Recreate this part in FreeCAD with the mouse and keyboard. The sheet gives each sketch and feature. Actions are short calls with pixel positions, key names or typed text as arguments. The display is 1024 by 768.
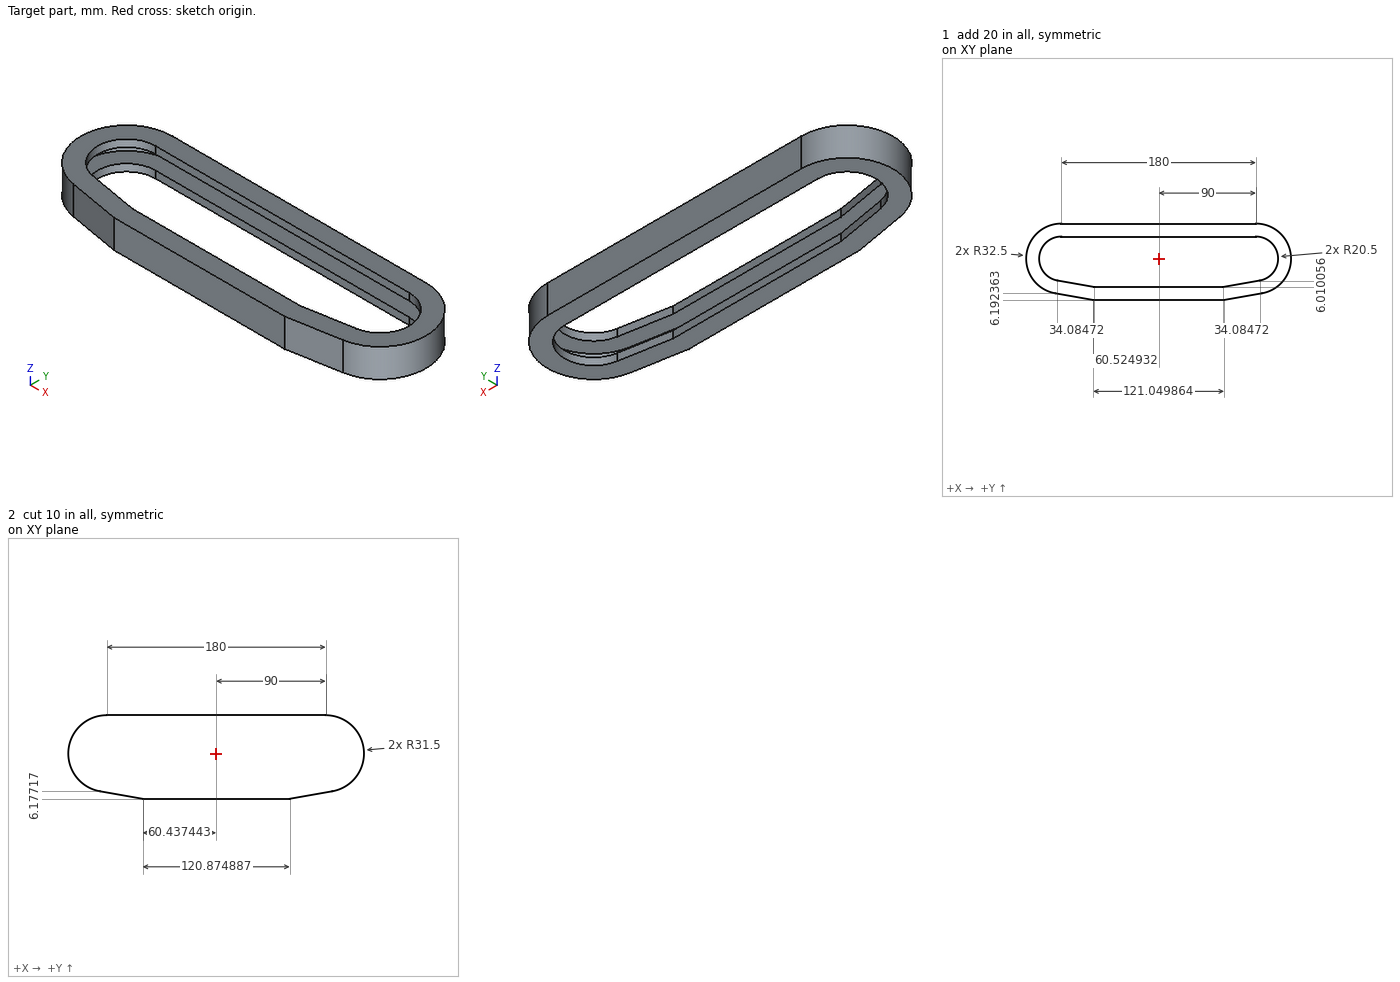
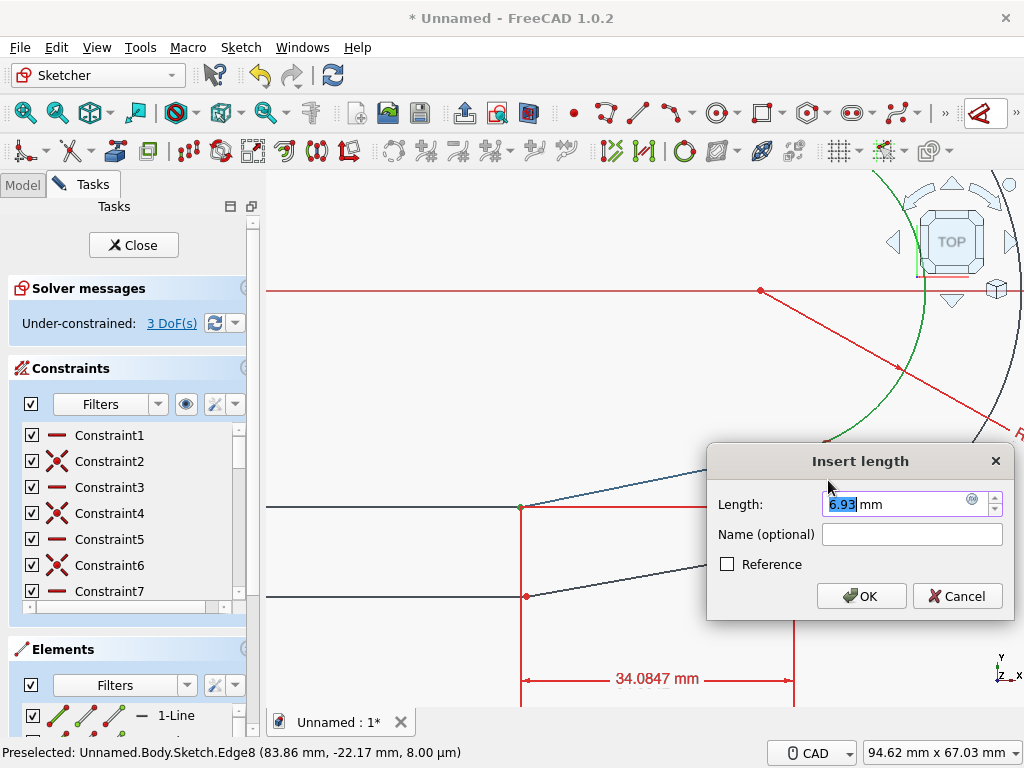
text(6.010056)
key(Return)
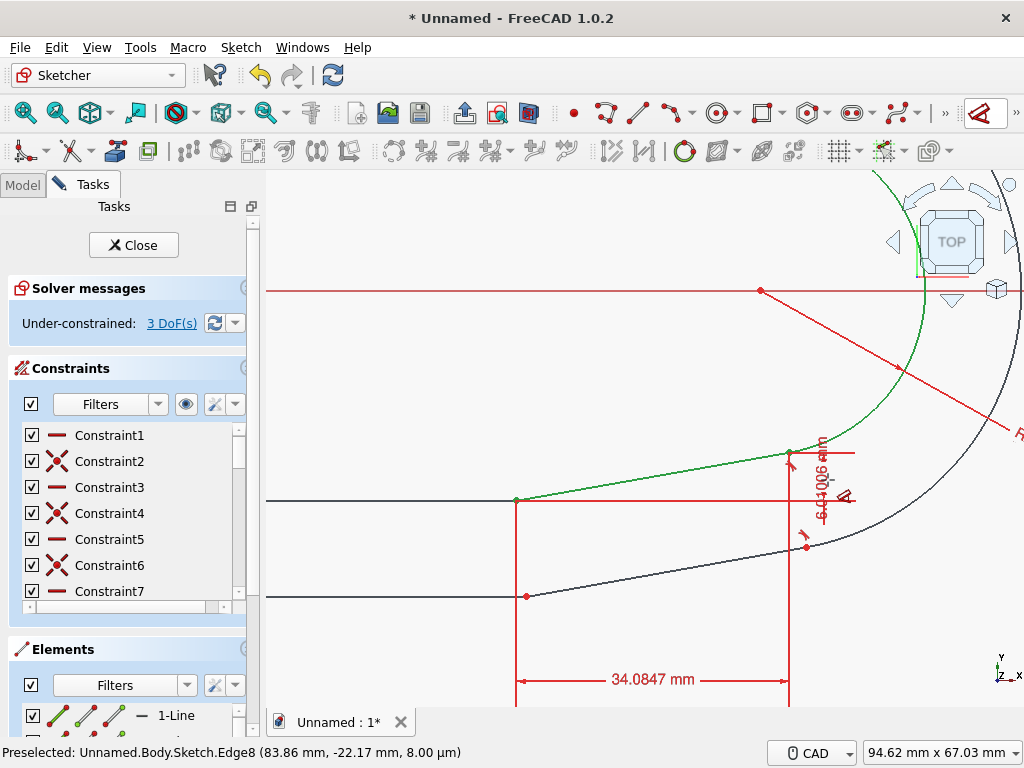
scroll(712, 470, down, 8)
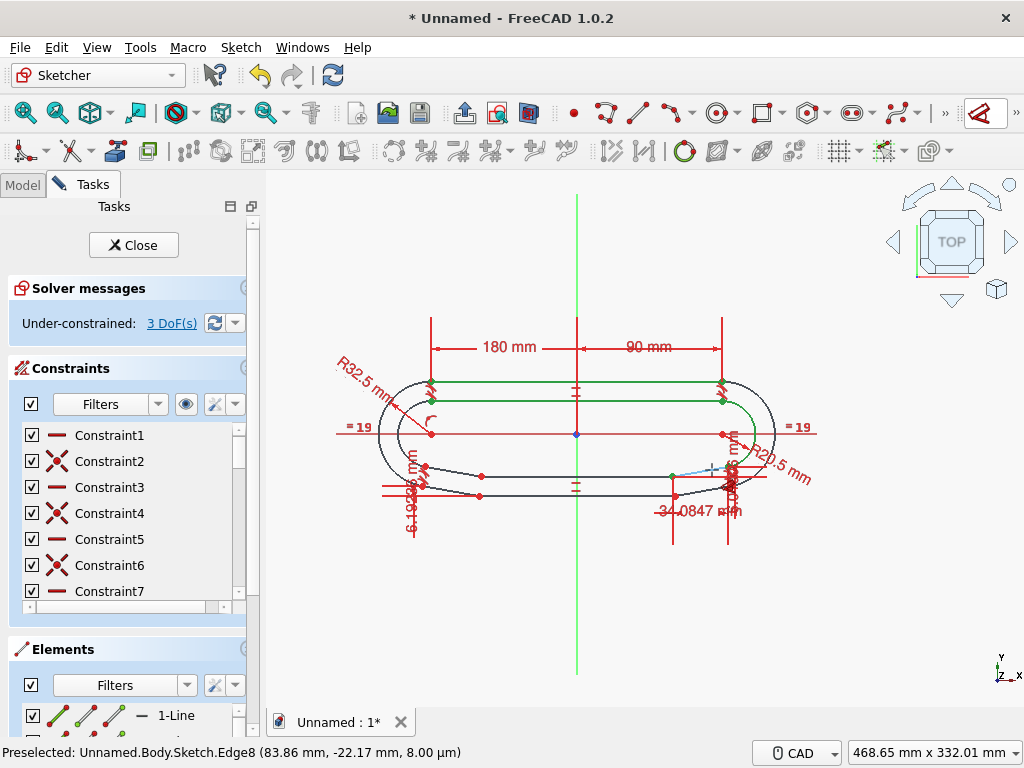
click(464, 474)
click(453, 535)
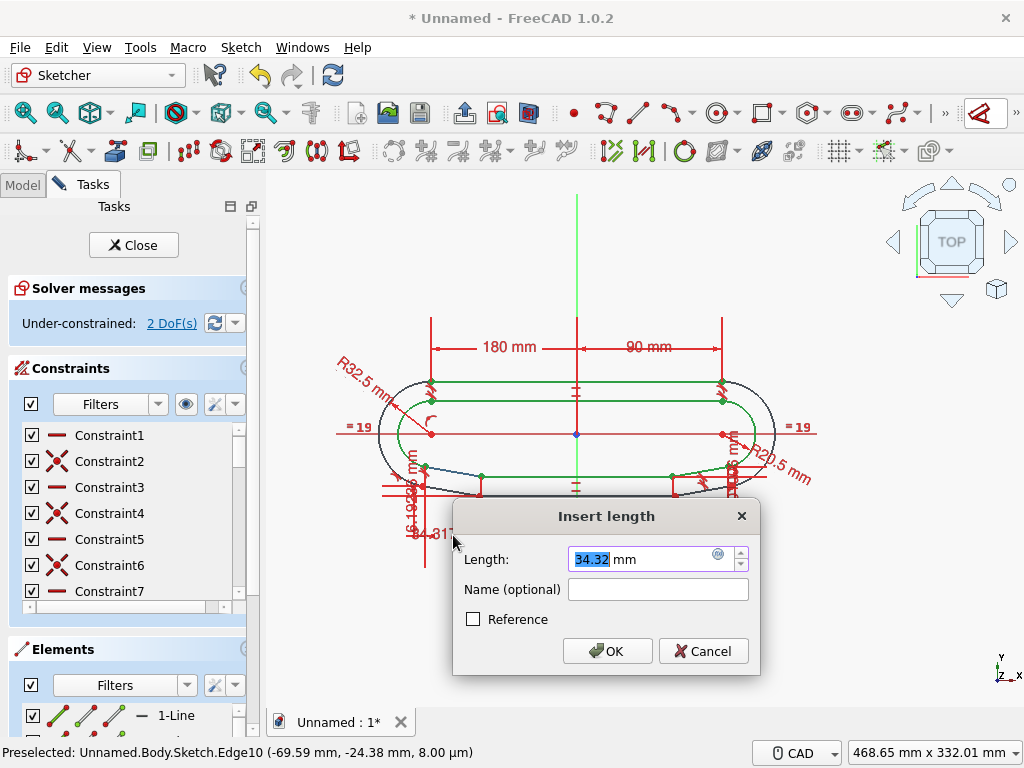
text(34.08472)
key(Return)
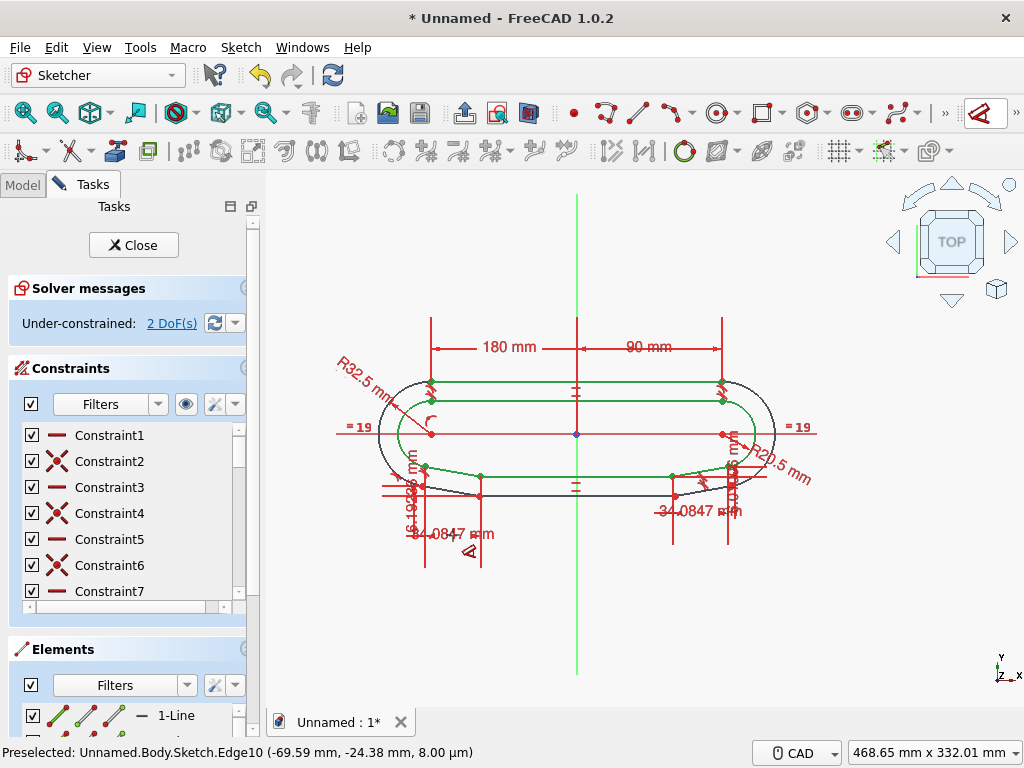
click(538, 496)
click(532, 530)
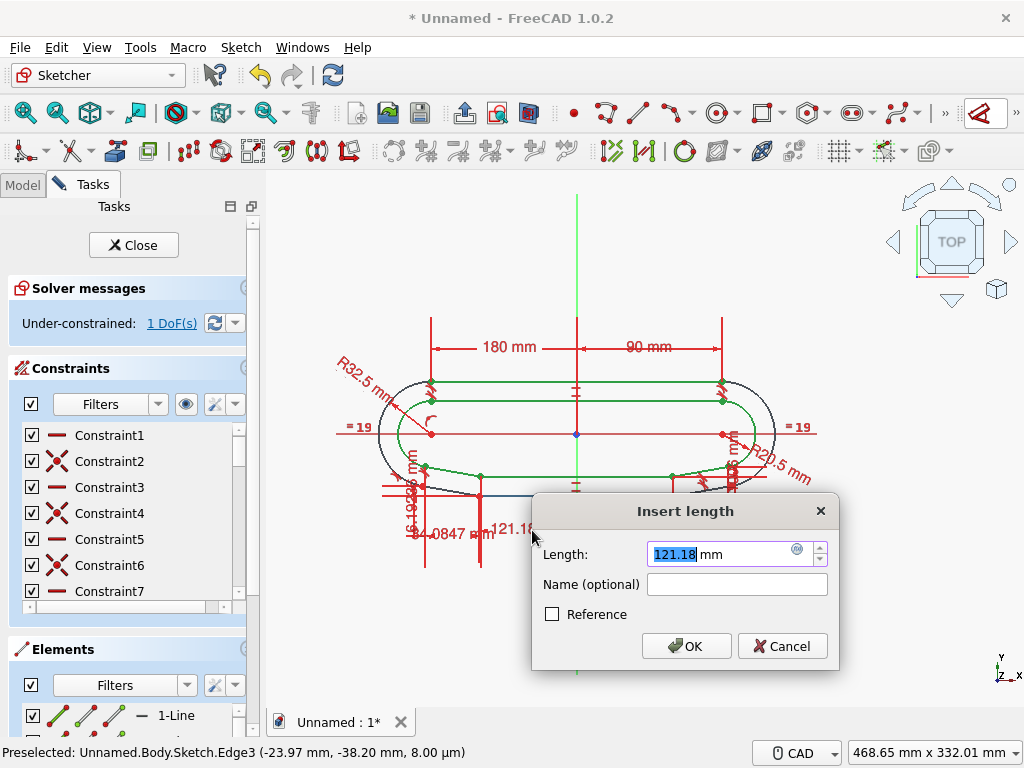
text(121.049864)
key(Return)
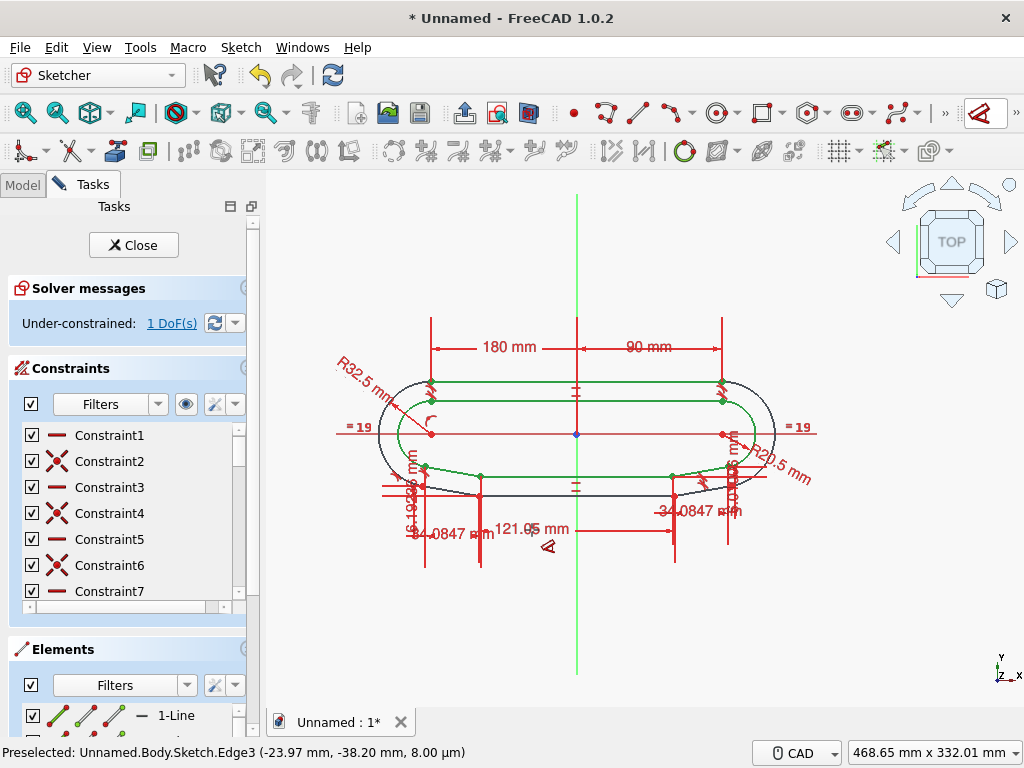
click(479, 496)
click(528, 554)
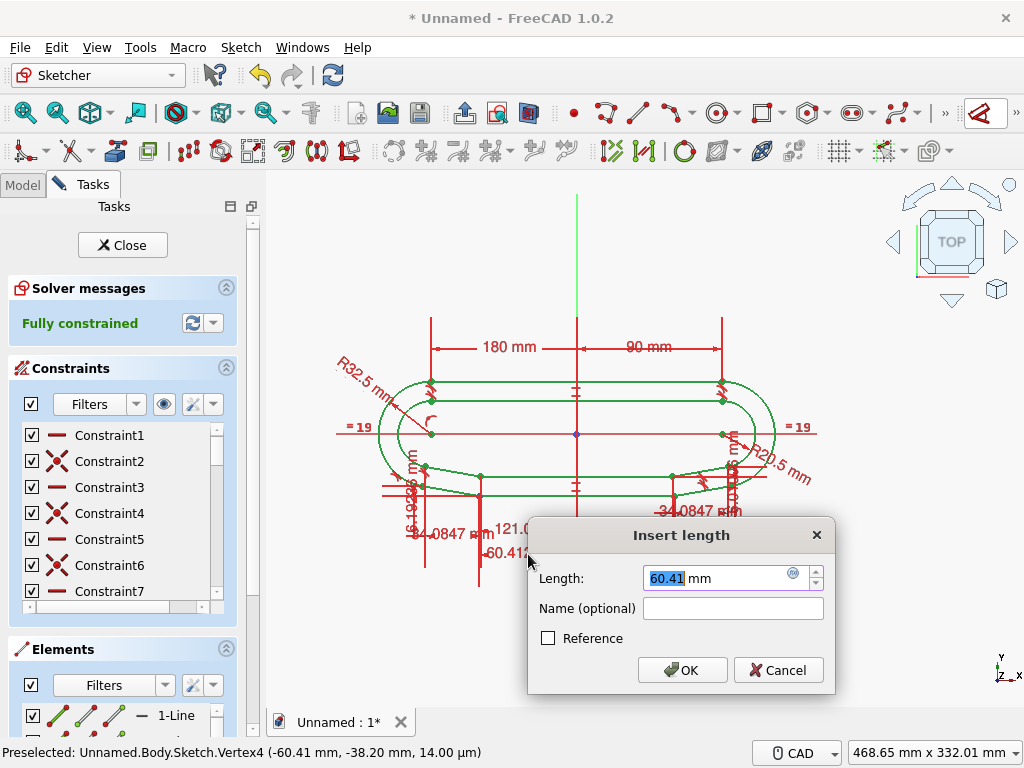
text(60.524932)
key(Return)
key(Escape)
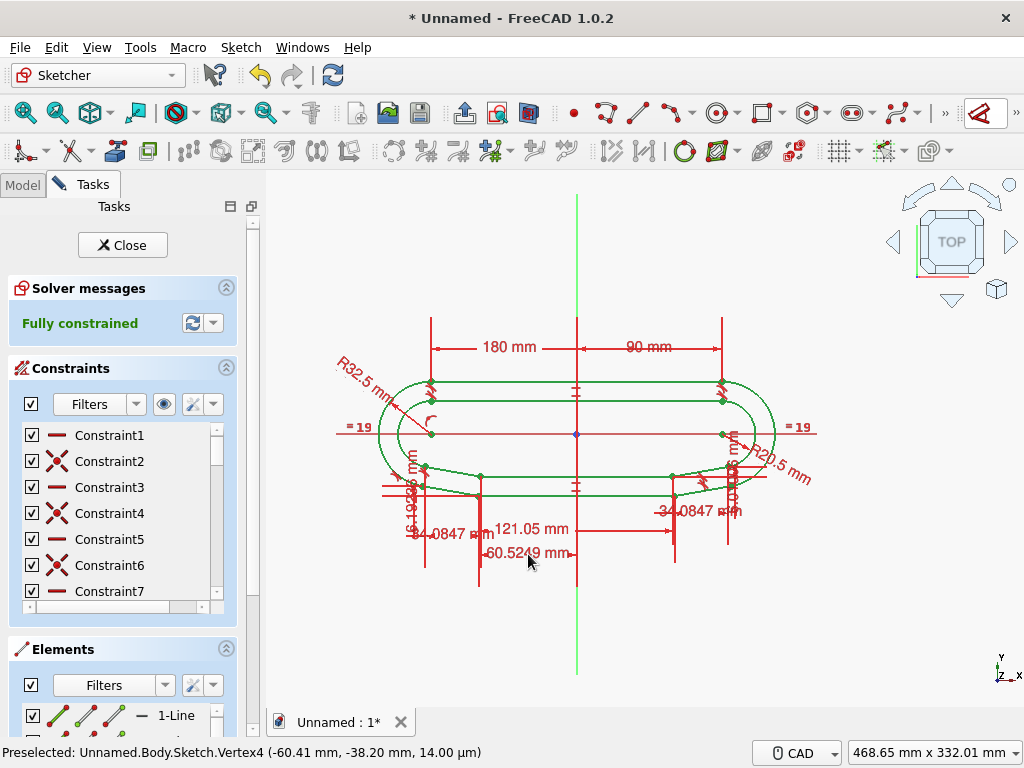
click(123, 245)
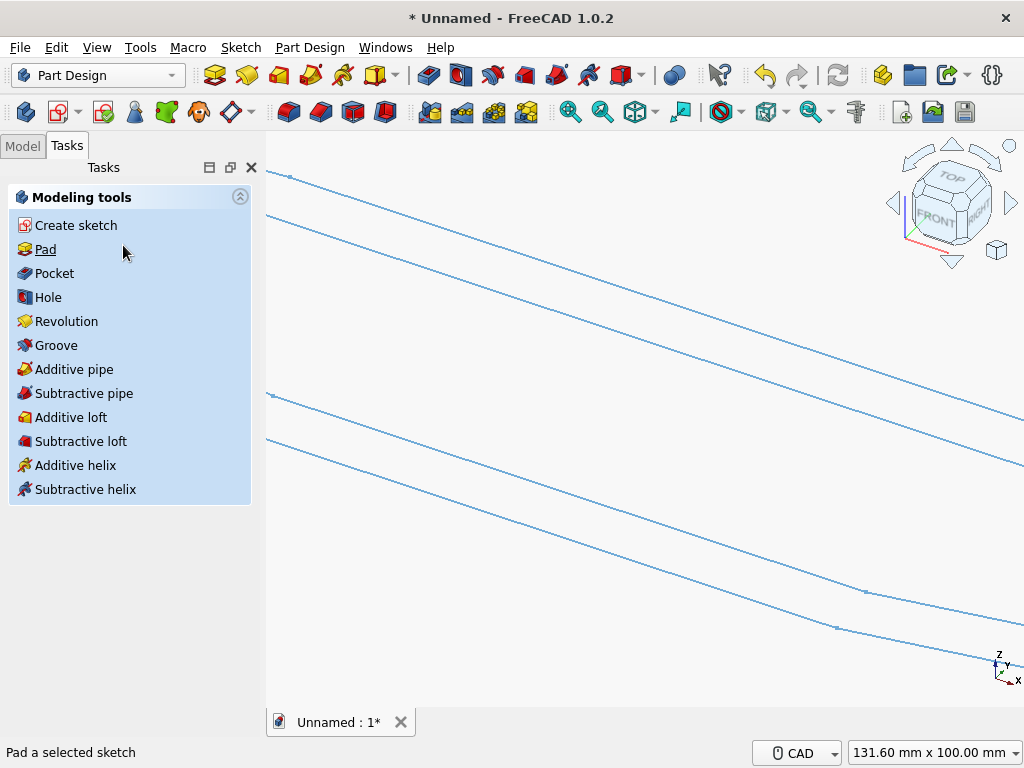
click(216, 76)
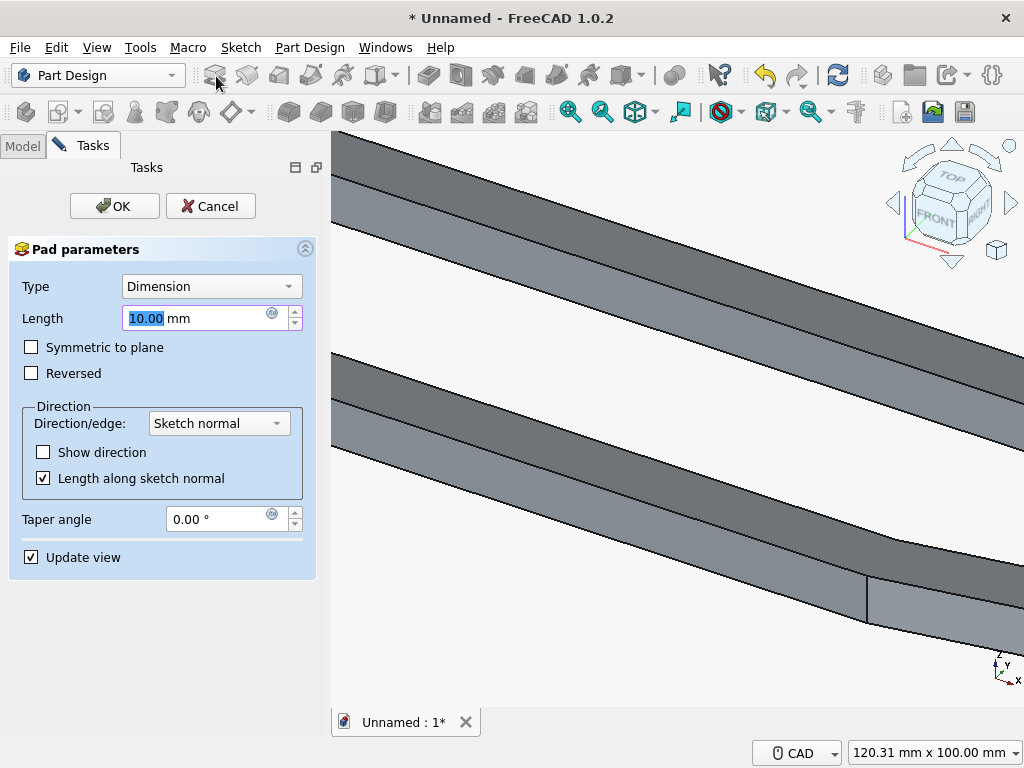
text(20)
key(Tab)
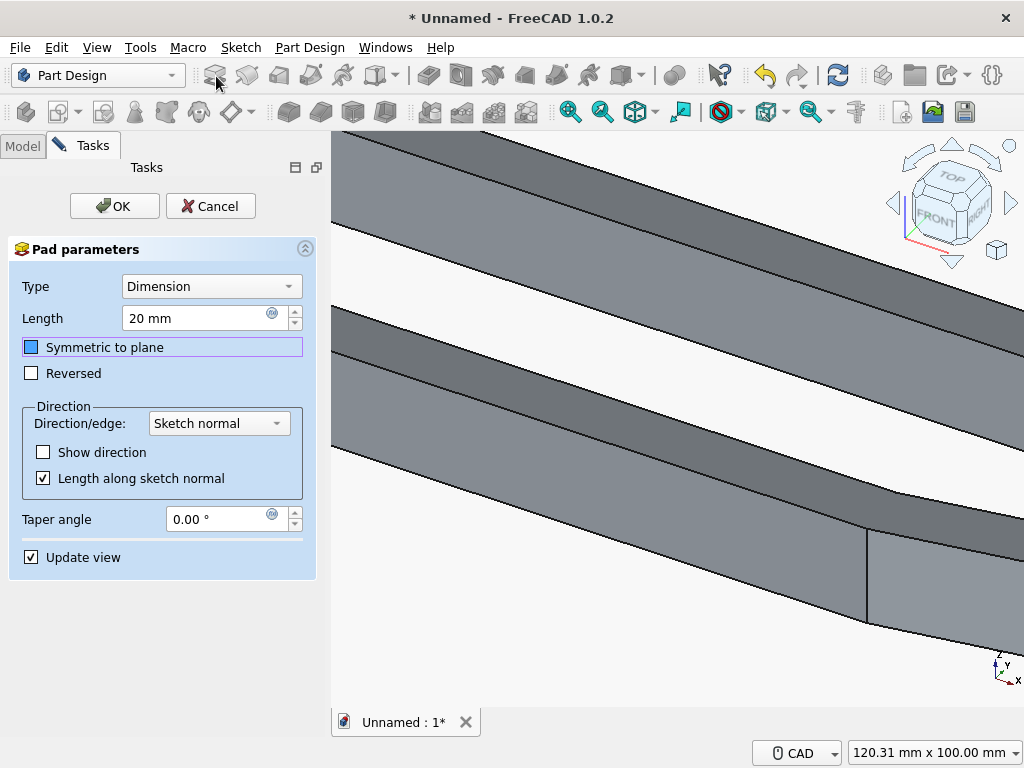
click(30, 347)